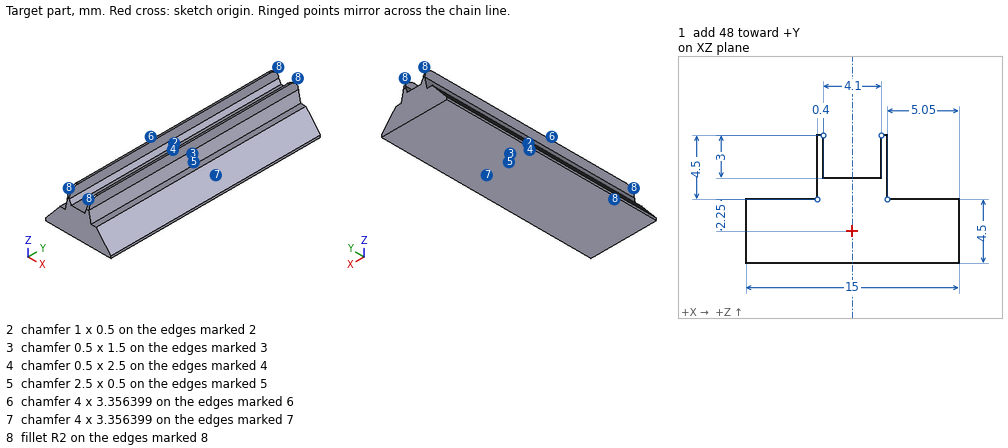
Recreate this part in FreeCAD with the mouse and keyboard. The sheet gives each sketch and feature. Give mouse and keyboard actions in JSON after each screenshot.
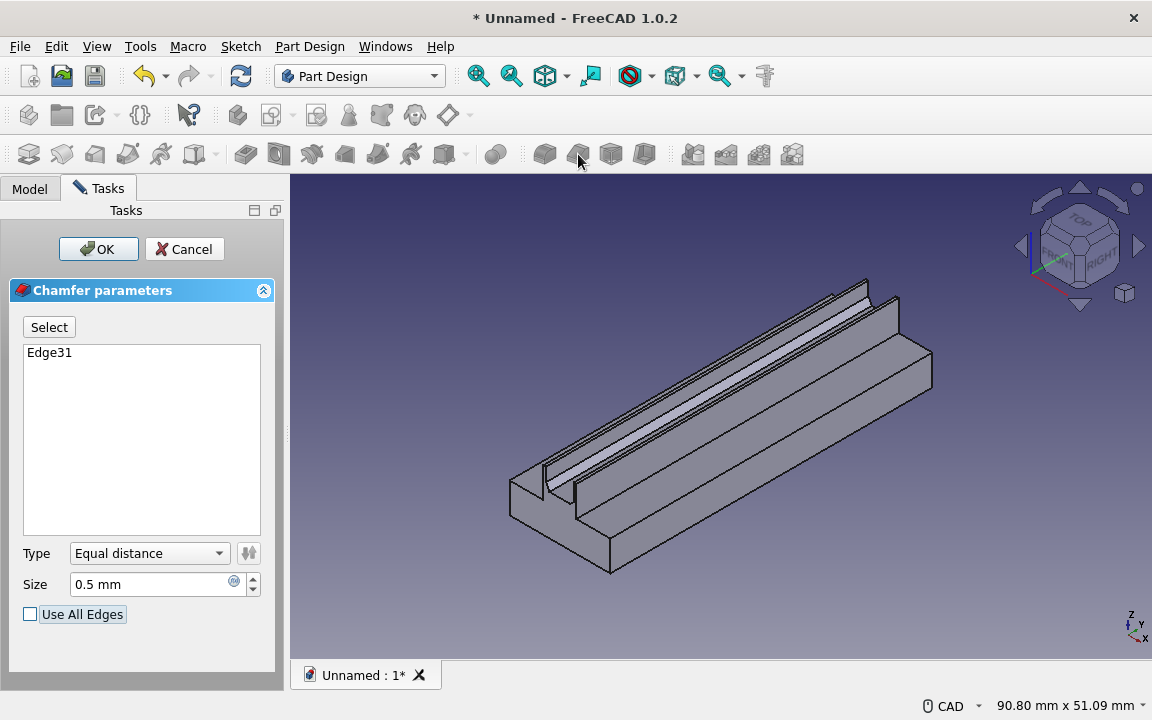
{"action": "left_click", "coordinate": [150, 554]}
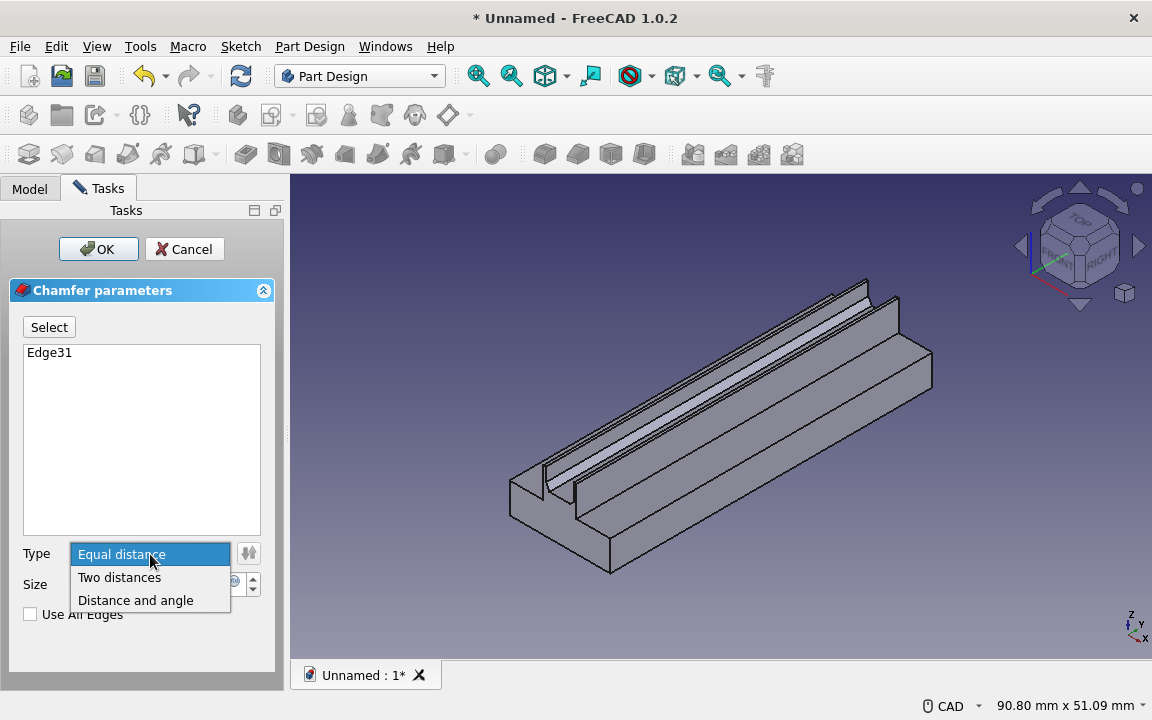
{"action": "left_click", "coordinate": [148, 578]}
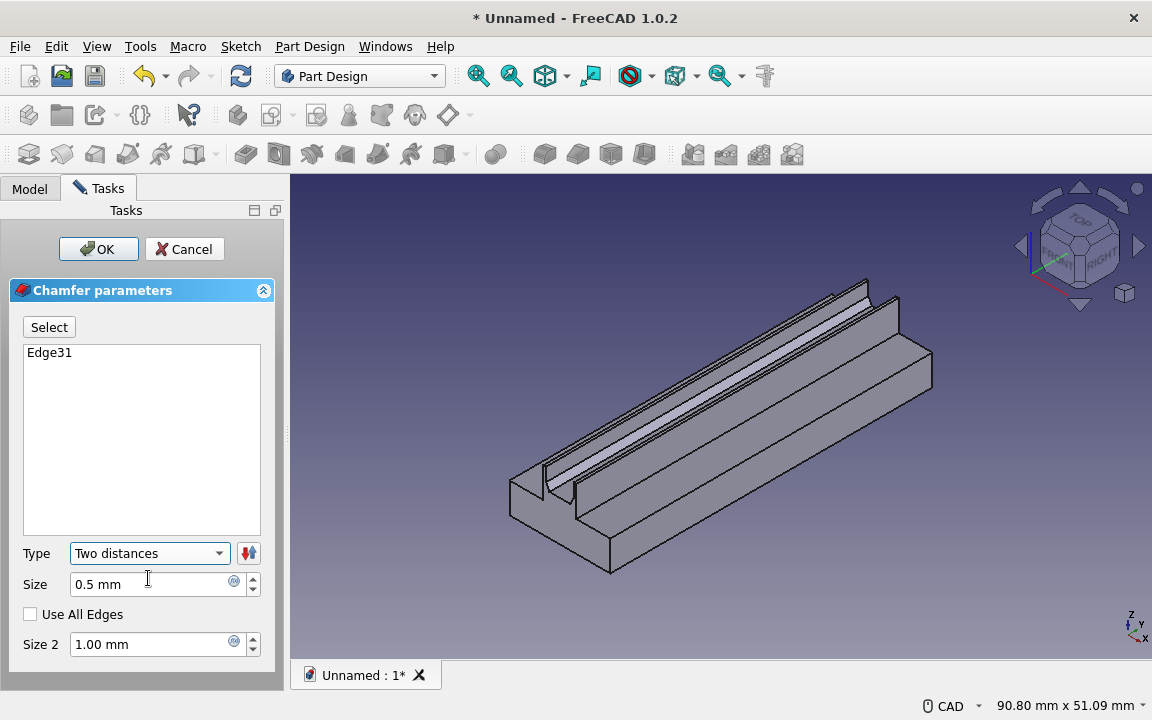
{"action": "triple_click", "coordinate": [158, 644]}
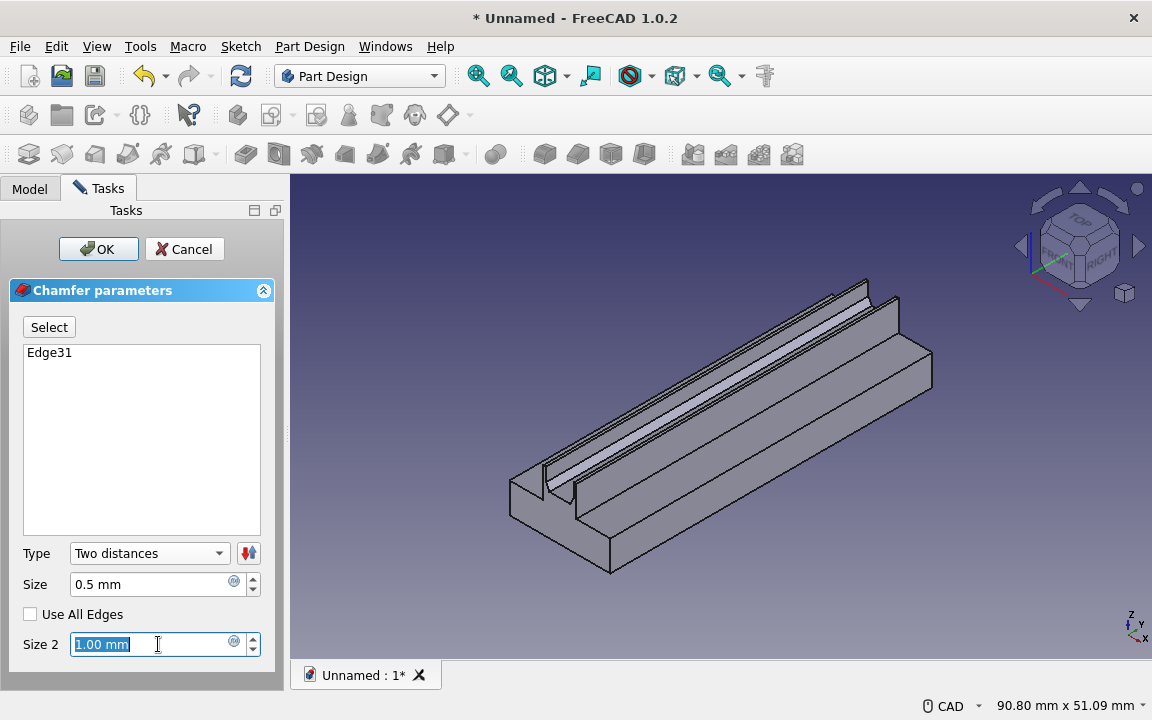
{"action": "type", "text": "1.5"}
{"action": "key", "text": "Tab"}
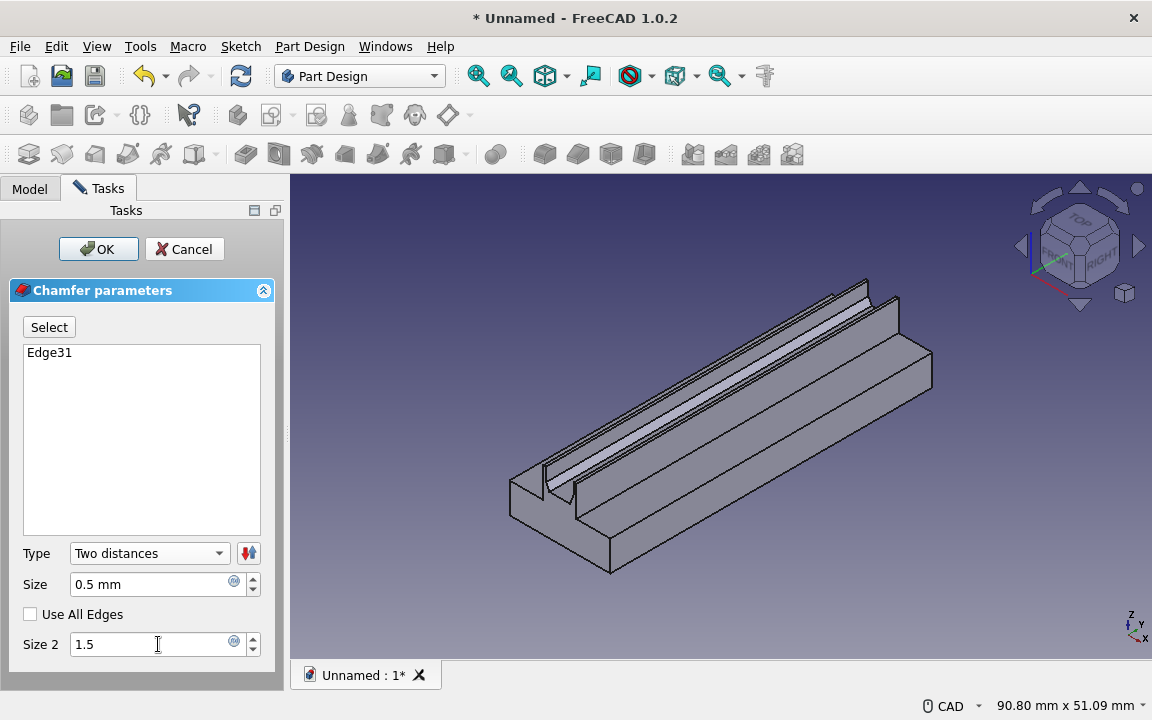
{"action": "left_click", "coordinate": [99, 249]}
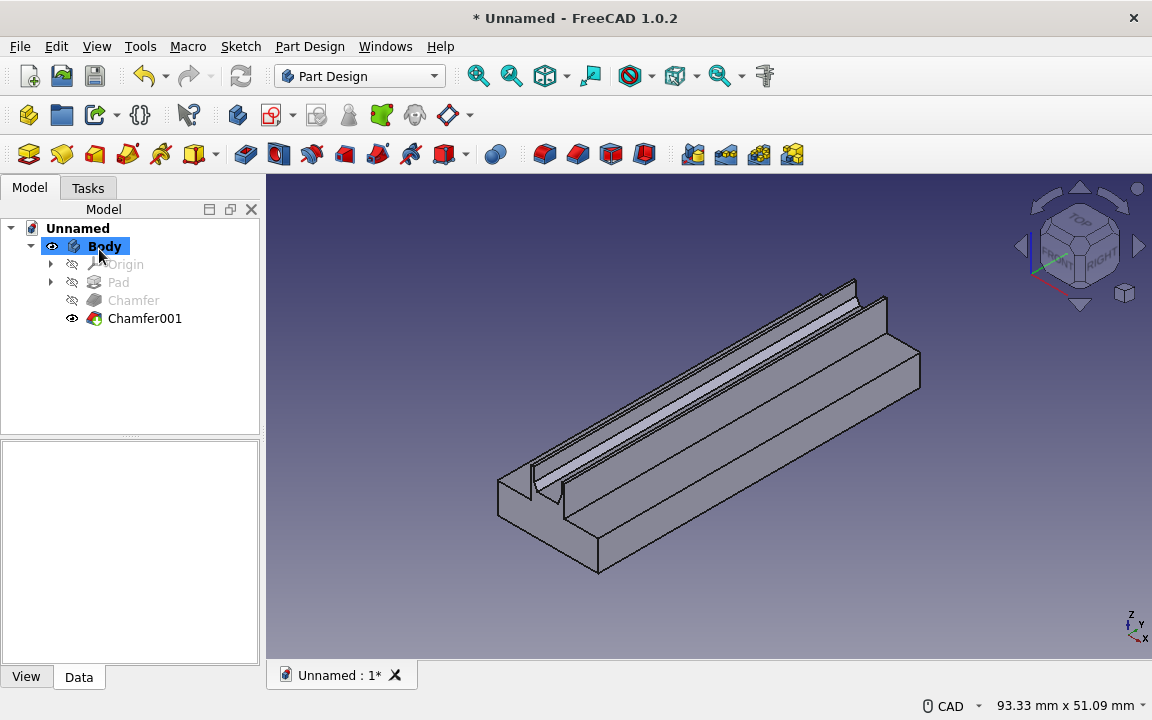
{"action": "key", "text": "2"}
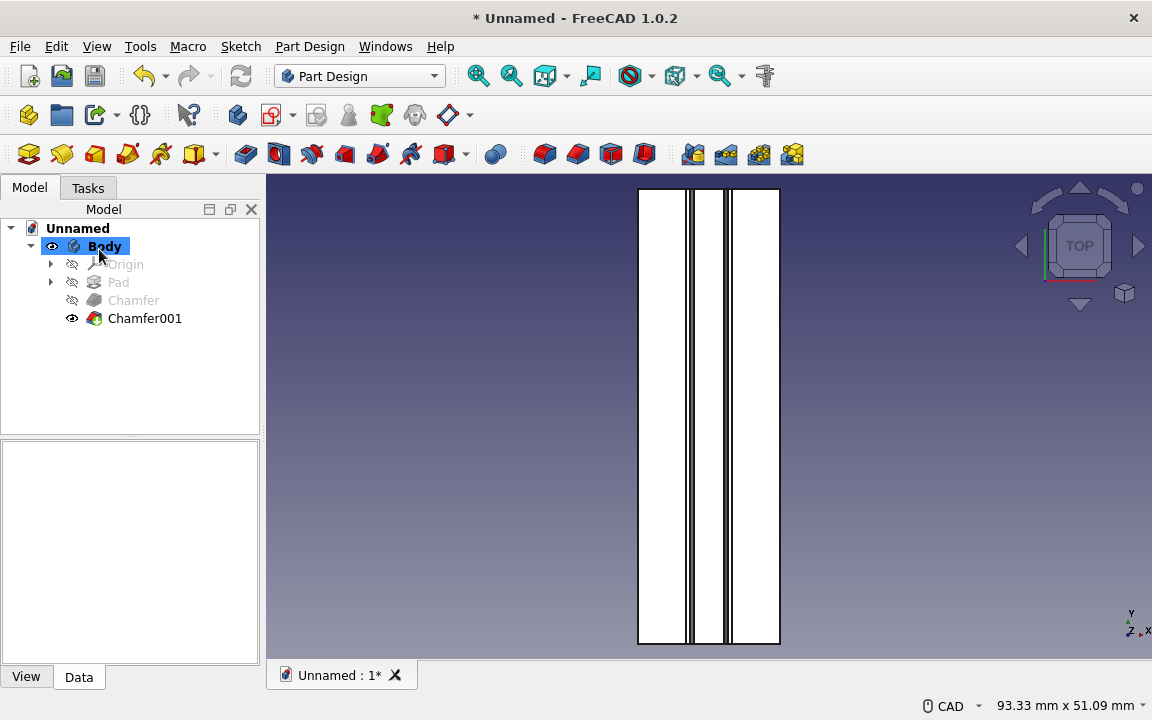
{"action": "key", "text": "0"}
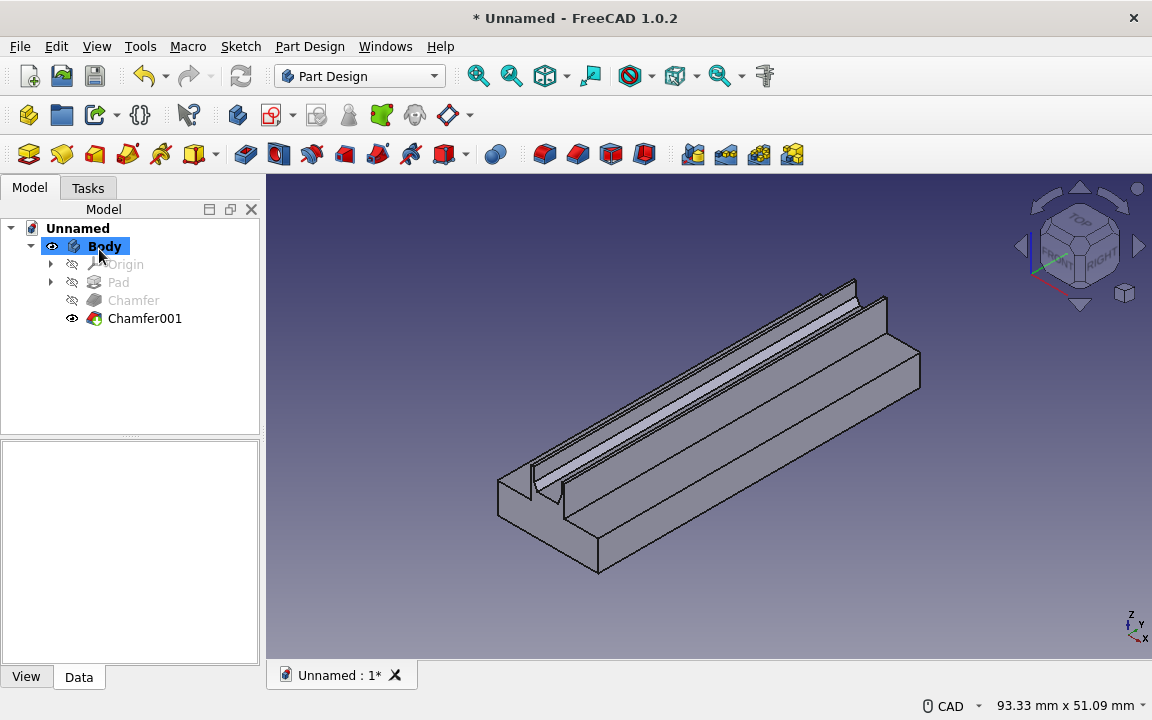
{"action": "key", "text": "1"}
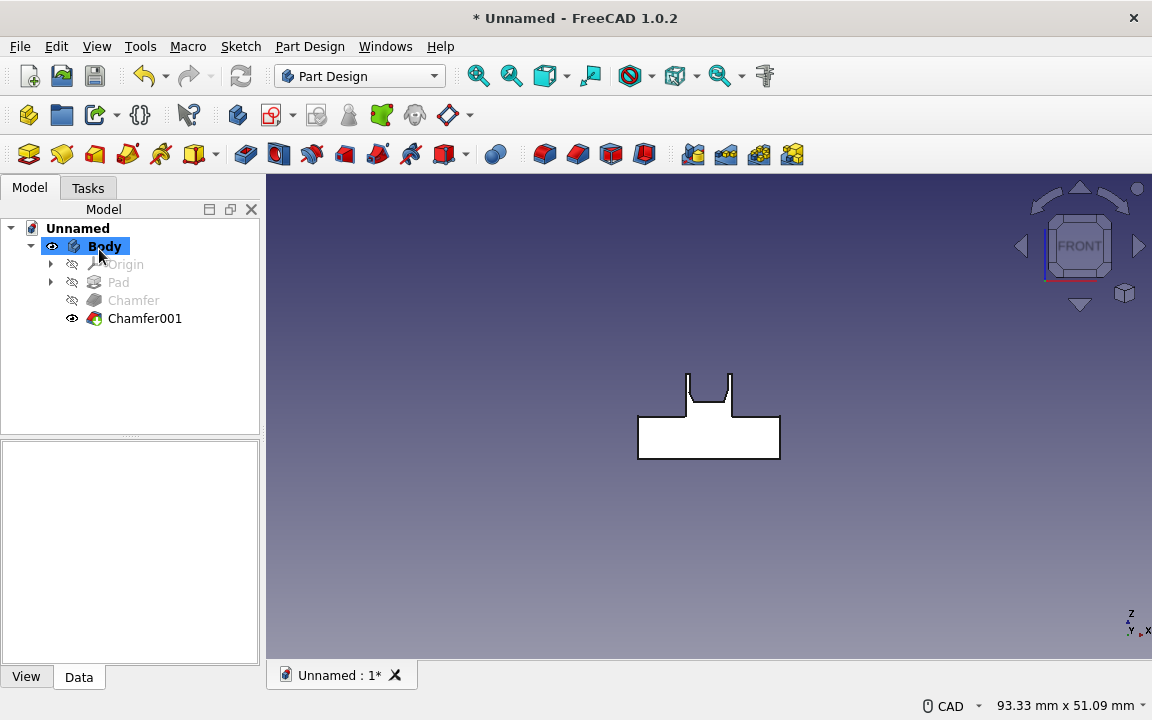
{"action": "left_click", "coordinate": [479, 76]}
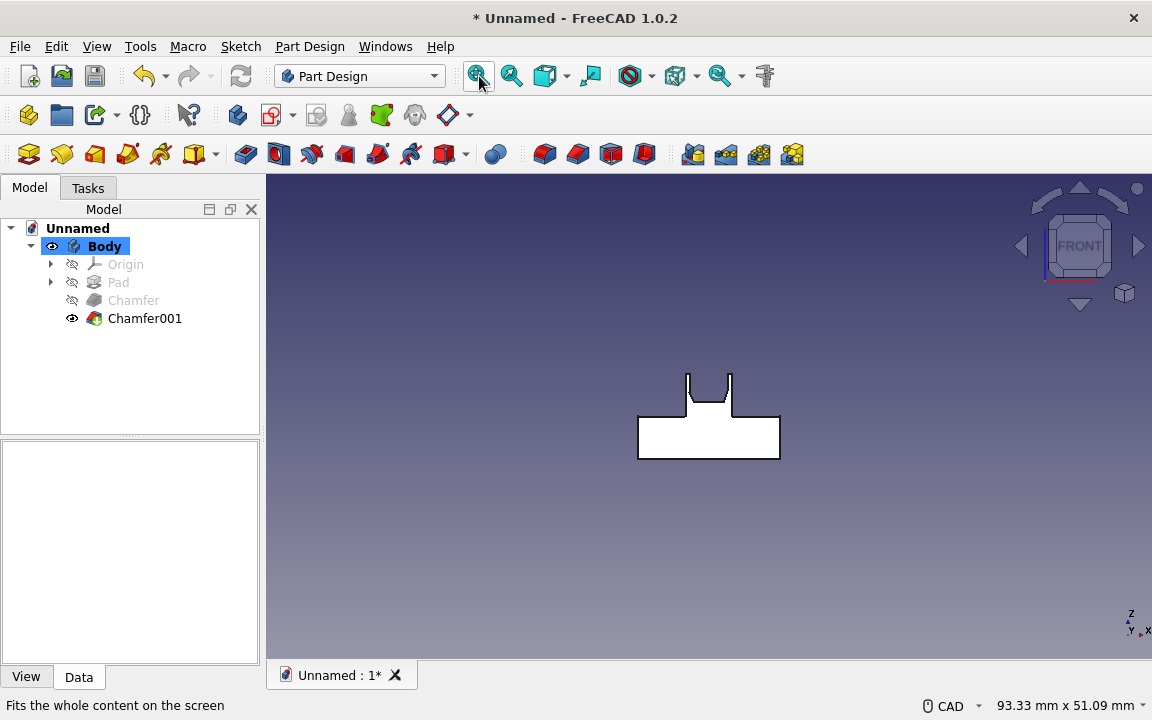
{"action": "key", "text": "3"}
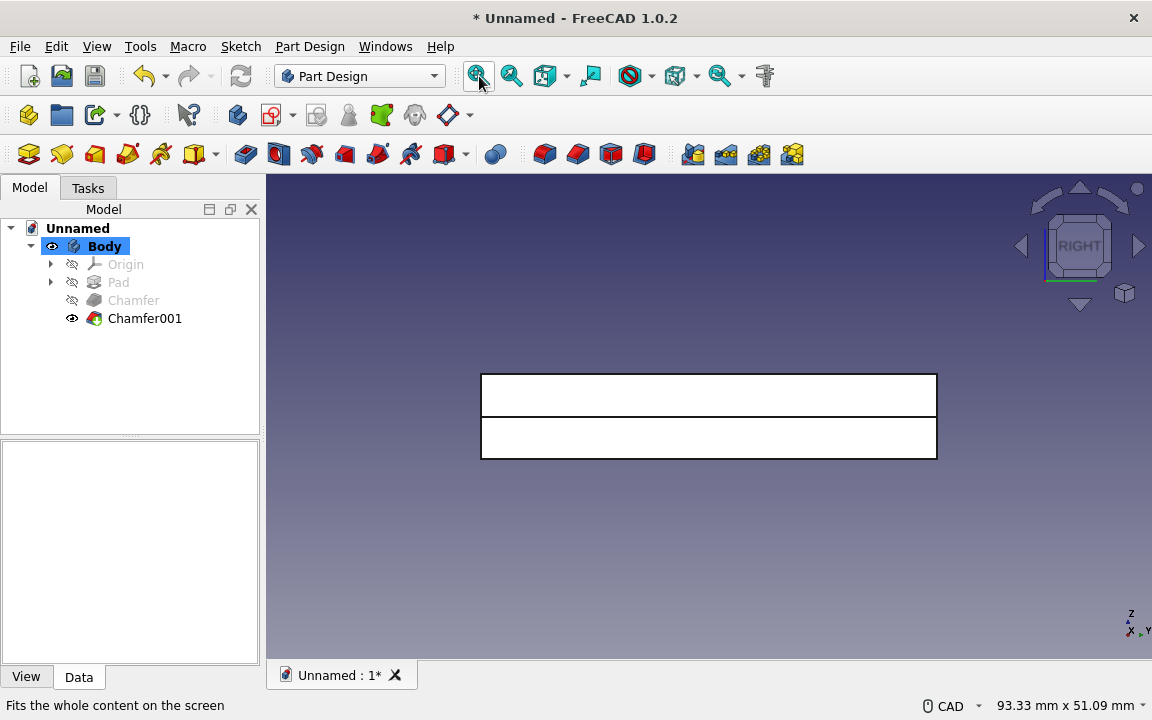
{"action": "key", "text": "5"}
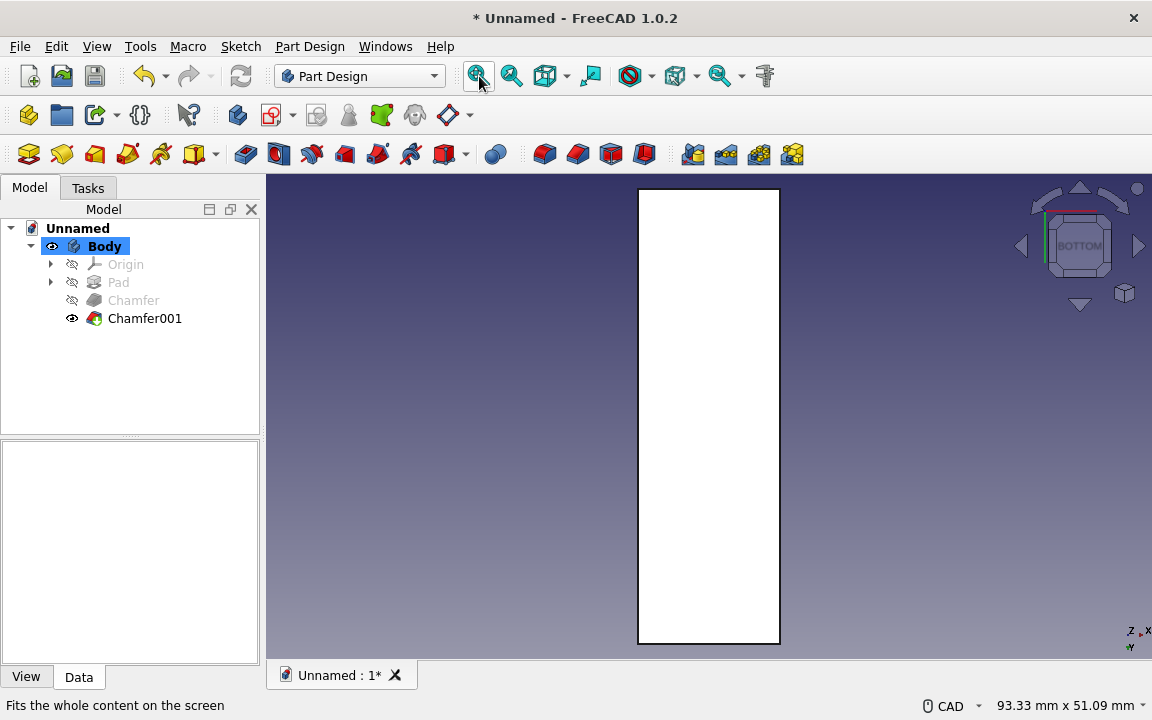
{"action": "key", "text": "4"}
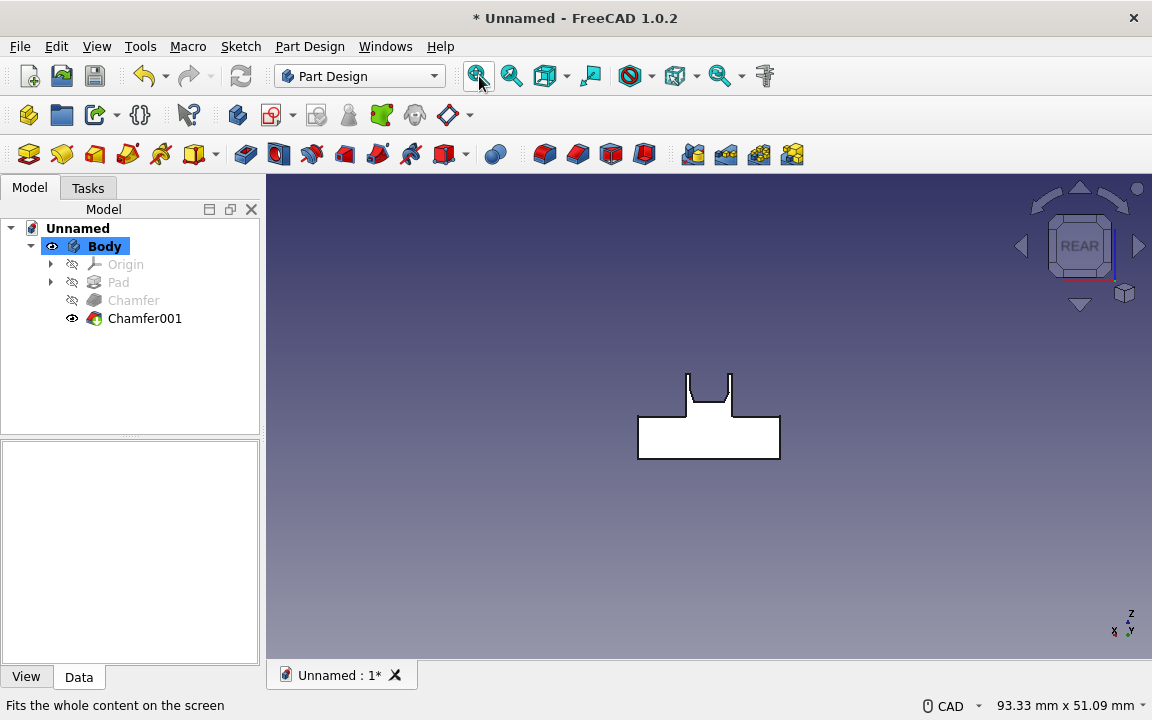
{"action": "left_click", "coordinate": [479, 76]}